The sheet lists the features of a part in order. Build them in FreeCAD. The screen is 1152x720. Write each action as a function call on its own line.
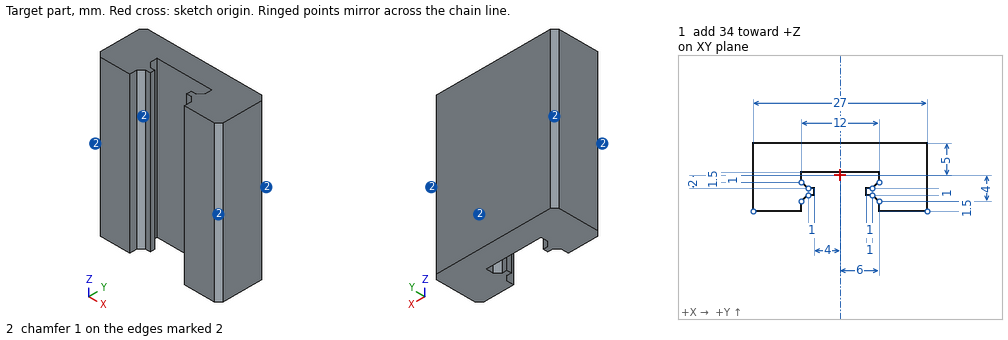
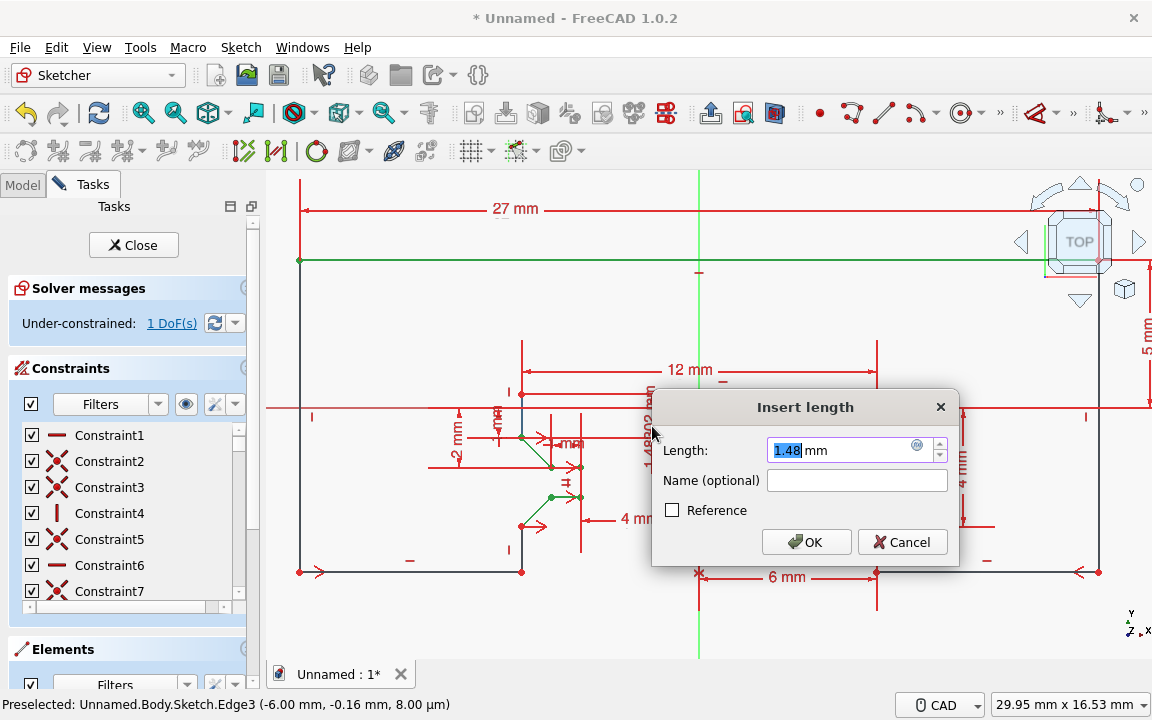
text(1.5)
key(Return)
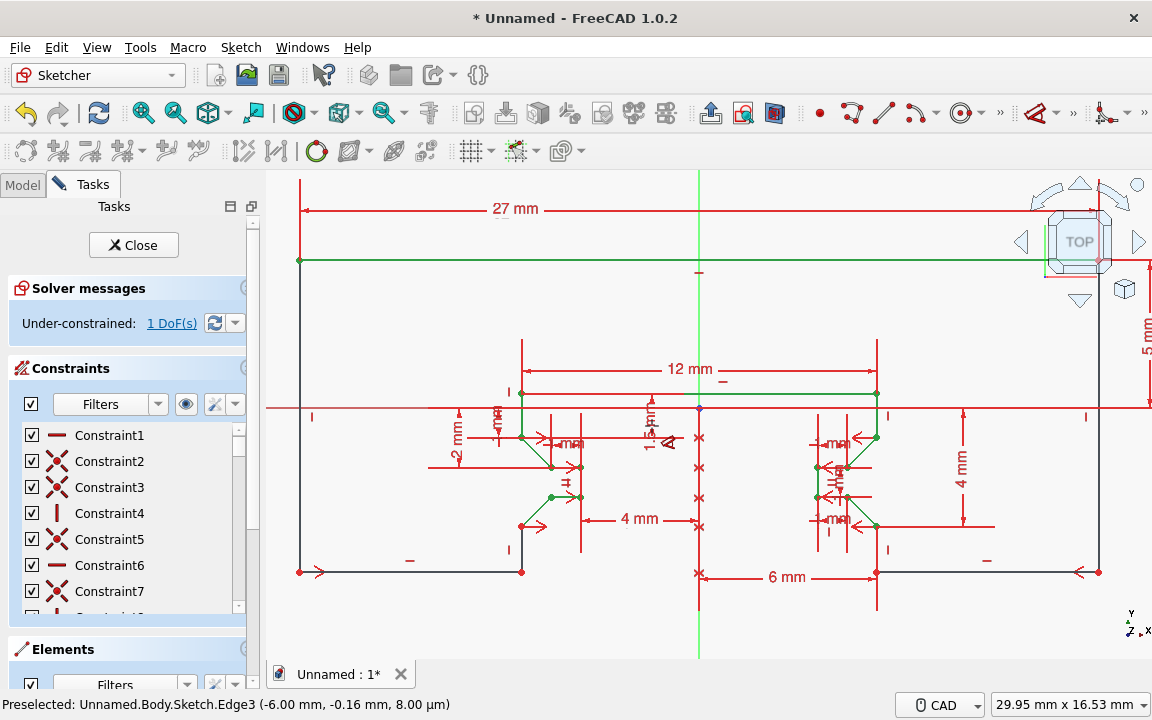
click(877, 540)
click(911, 549)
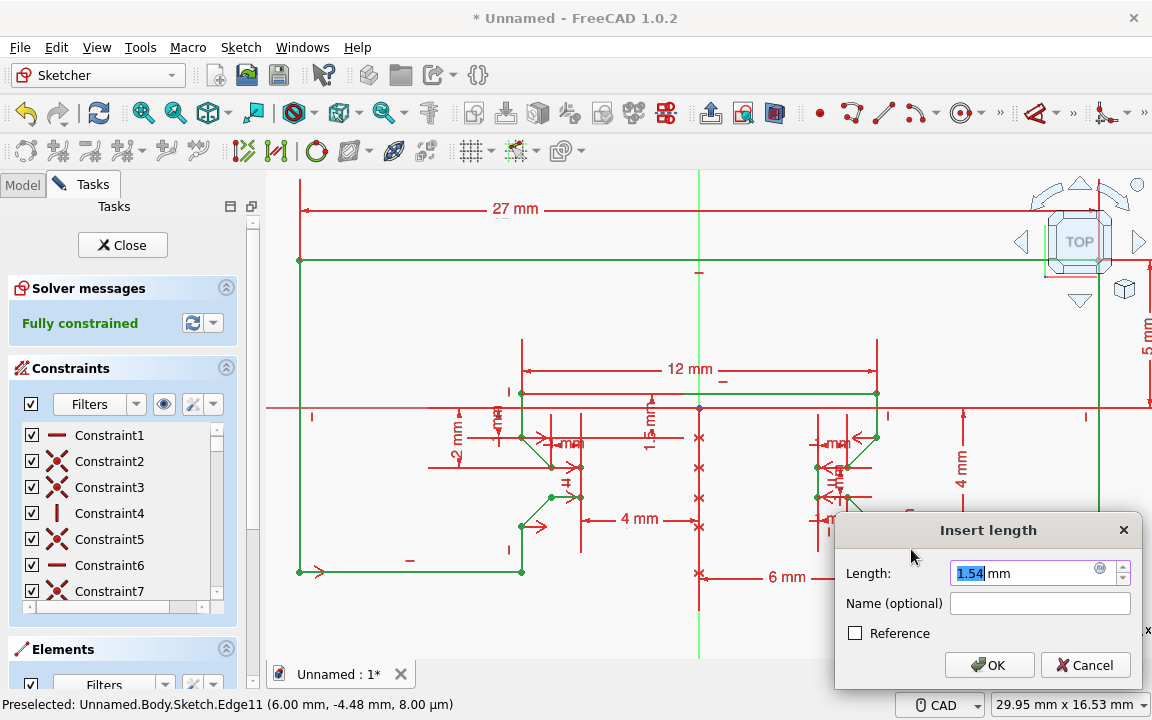
text(1.5)
key(Return)
key(Escape)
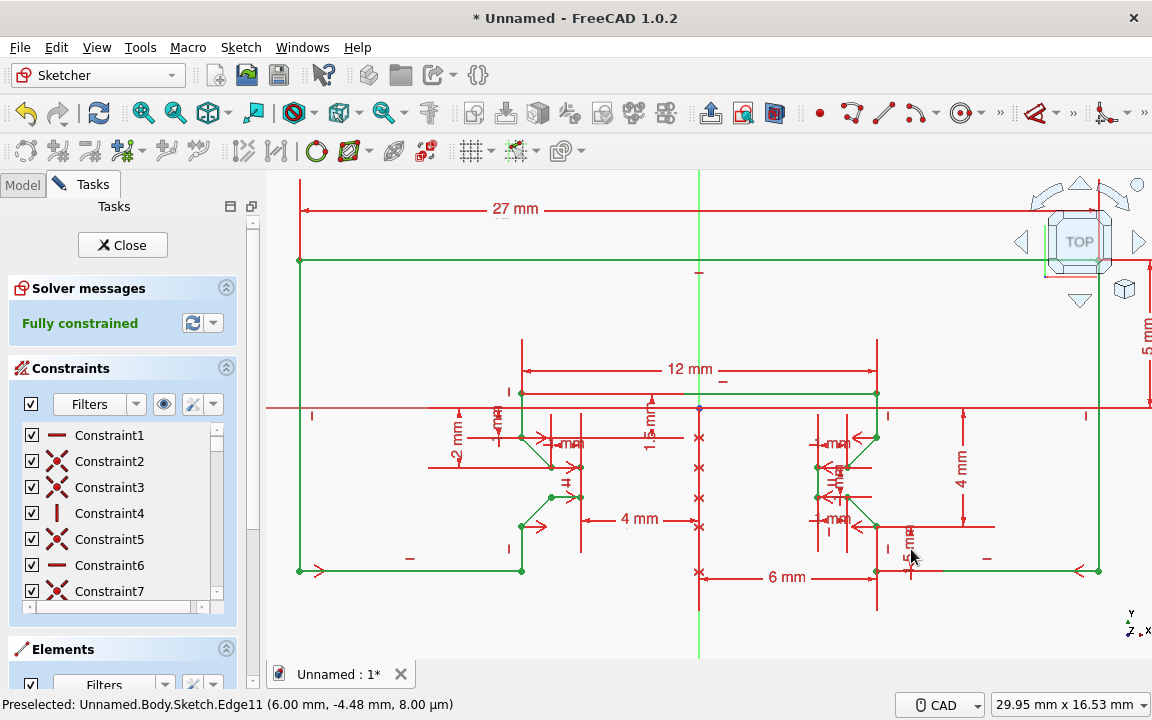
click(123, 245)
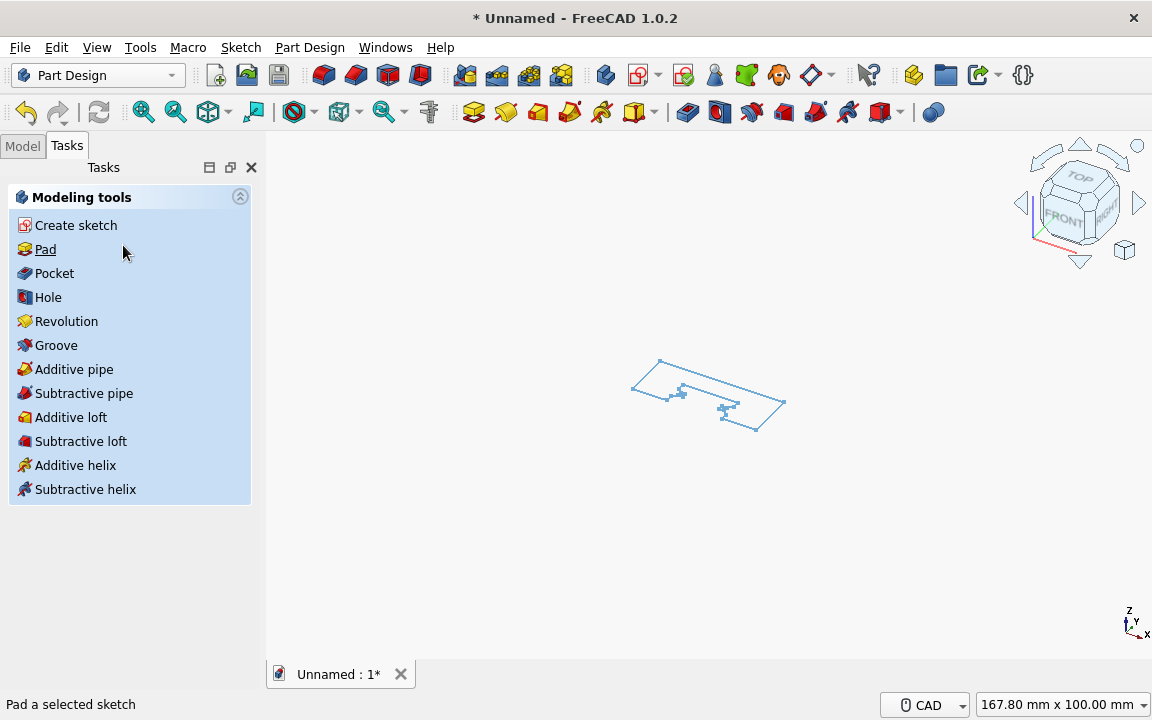
click(474, 112)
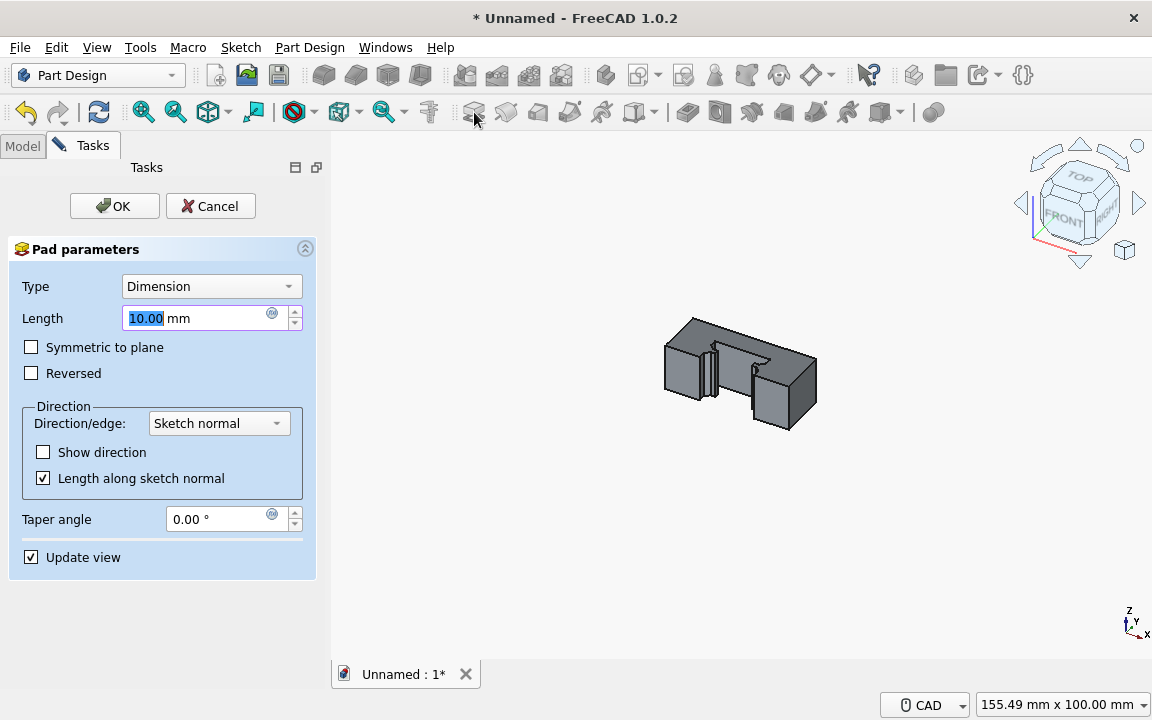
text(34)
key(Tab)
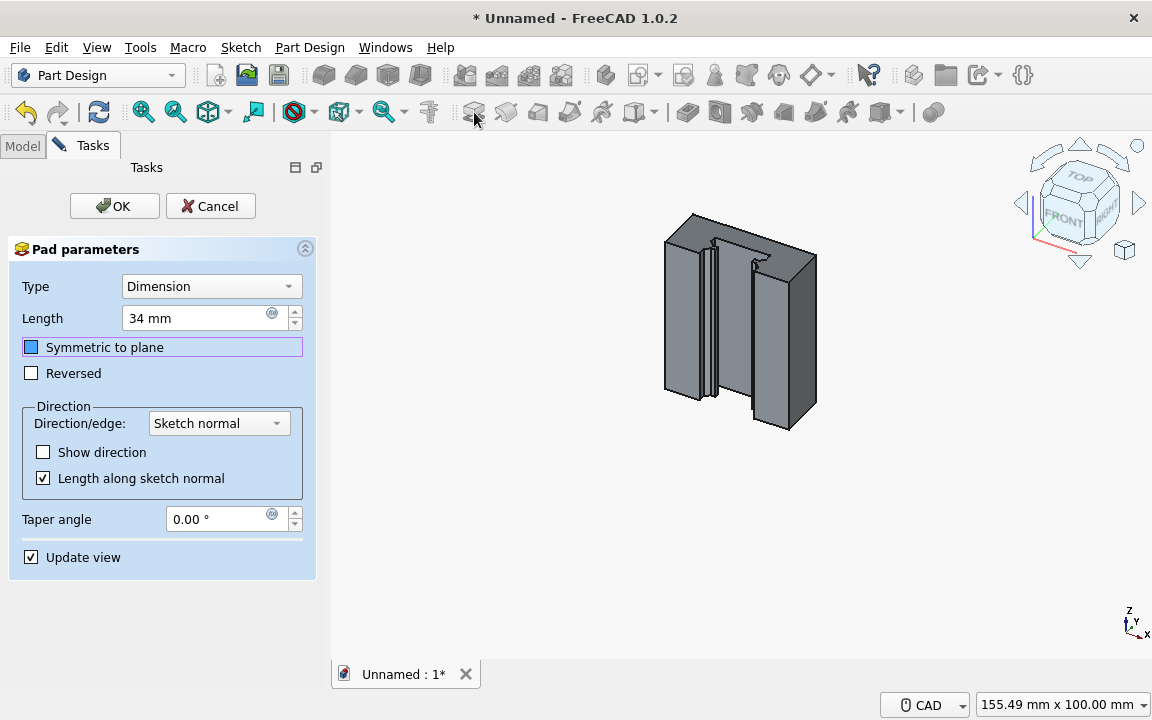
click(115, 206)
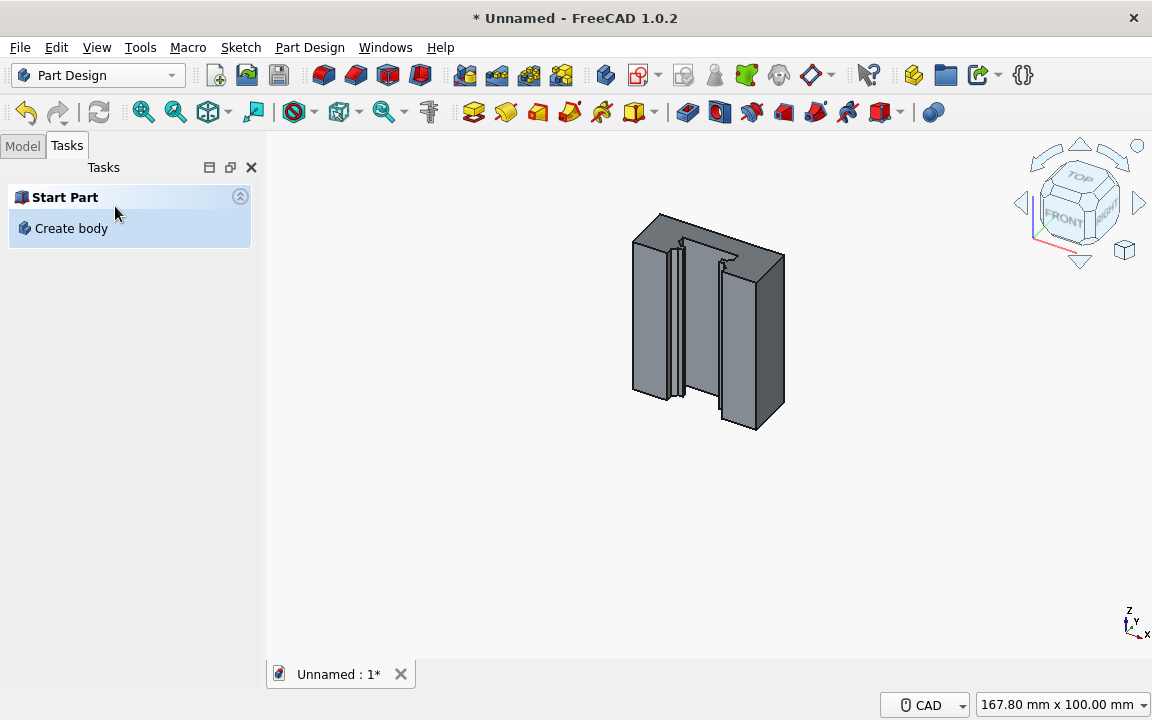
click(144, 112)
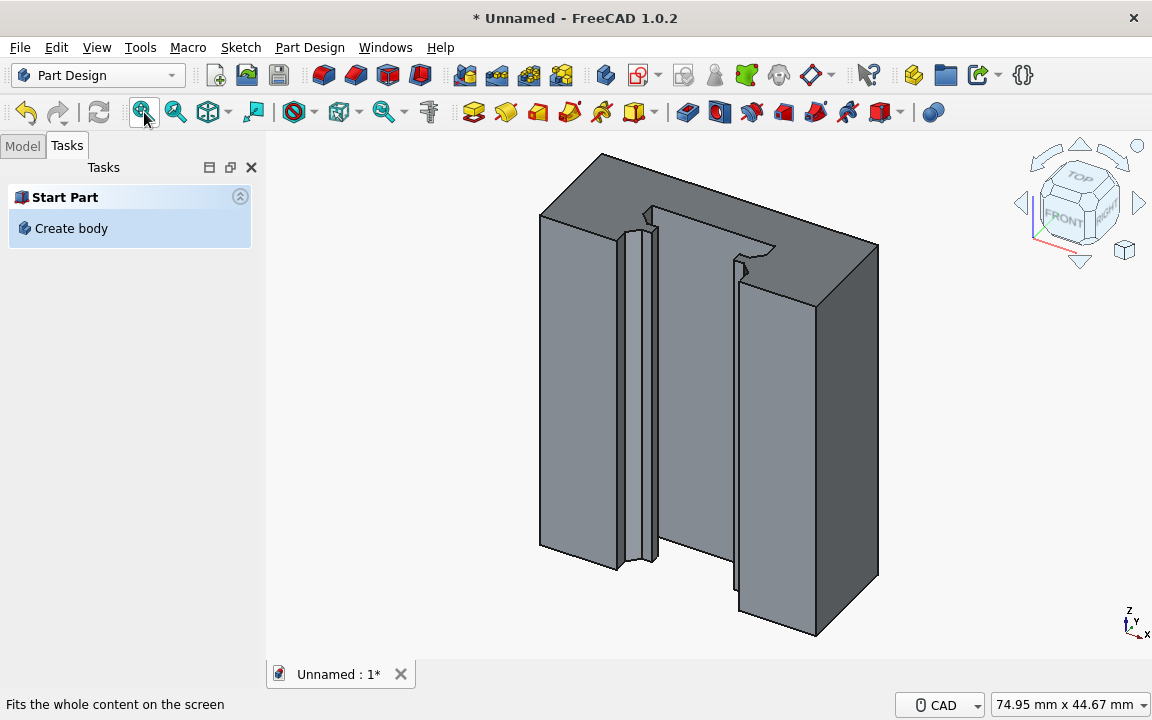
click(816, 471)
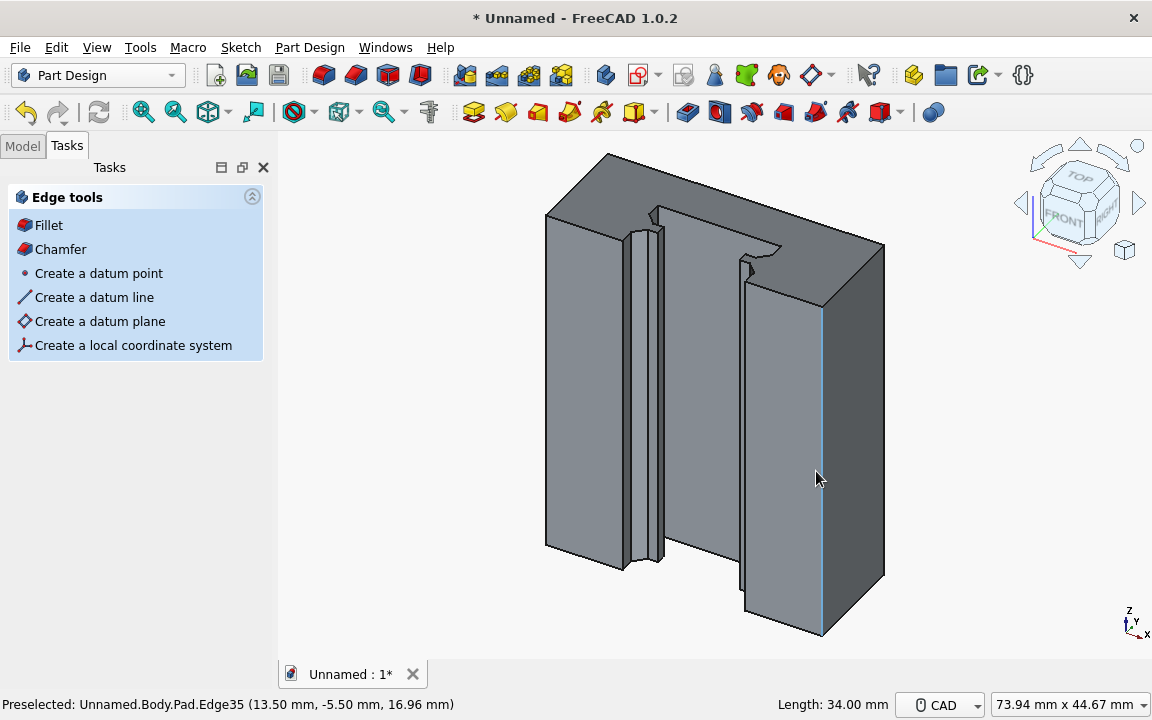
key(0)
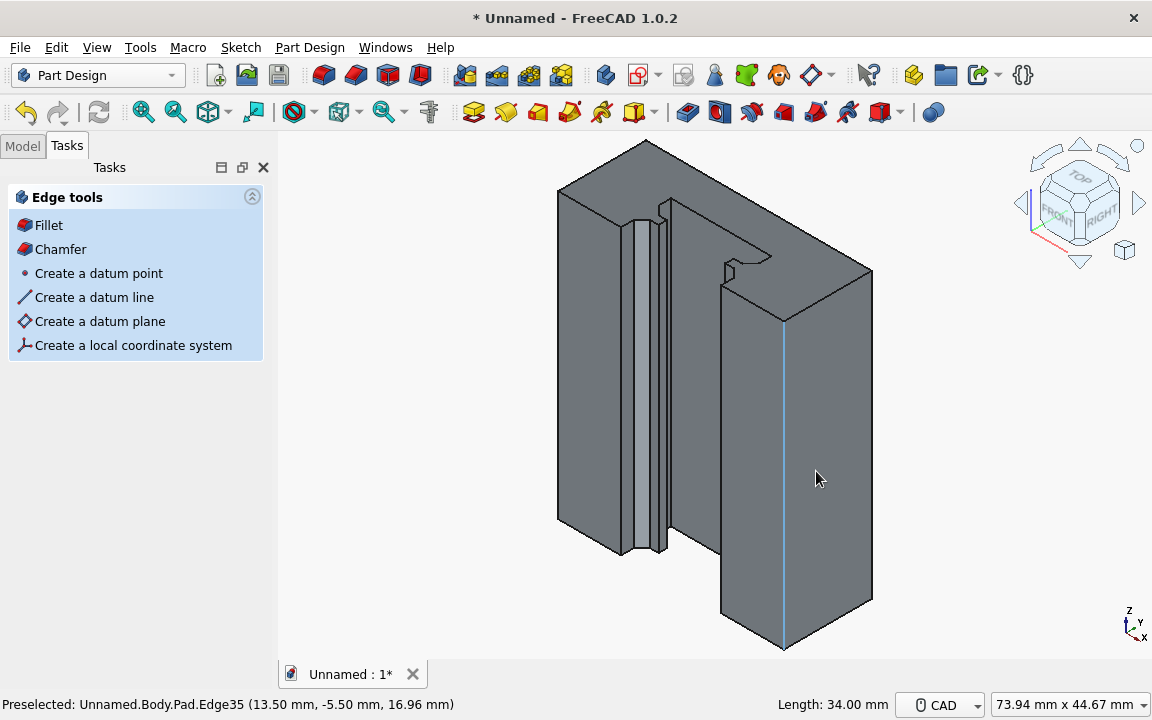
key(2)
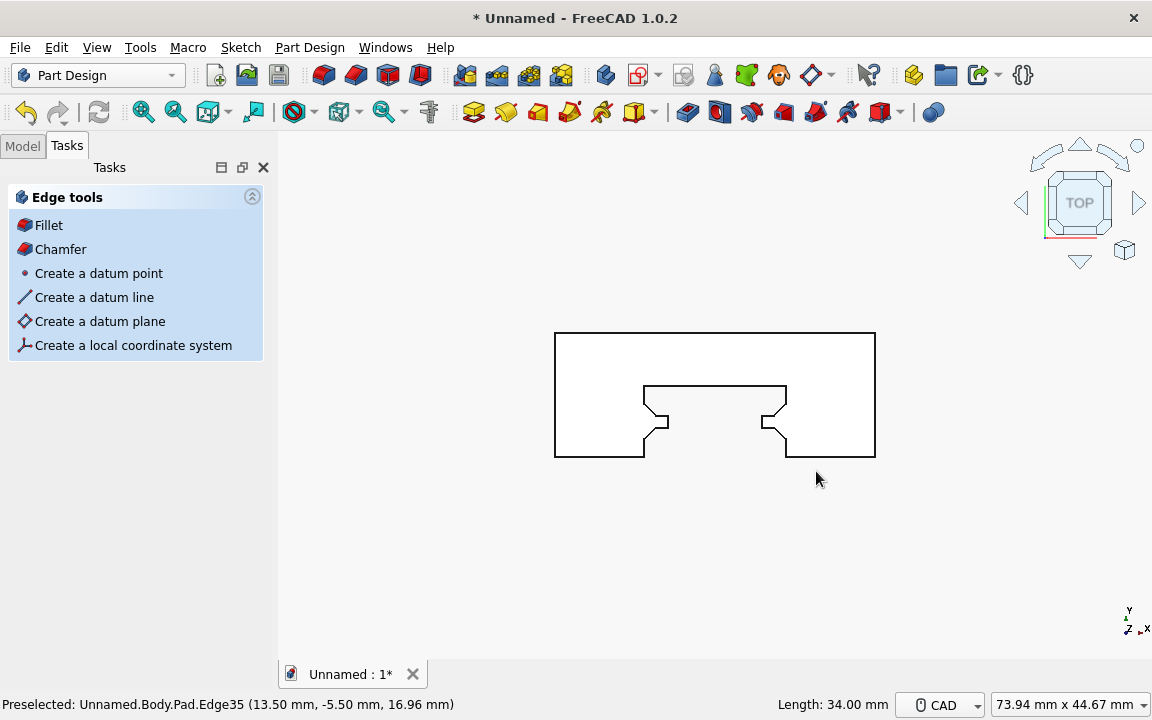
click(144, 112)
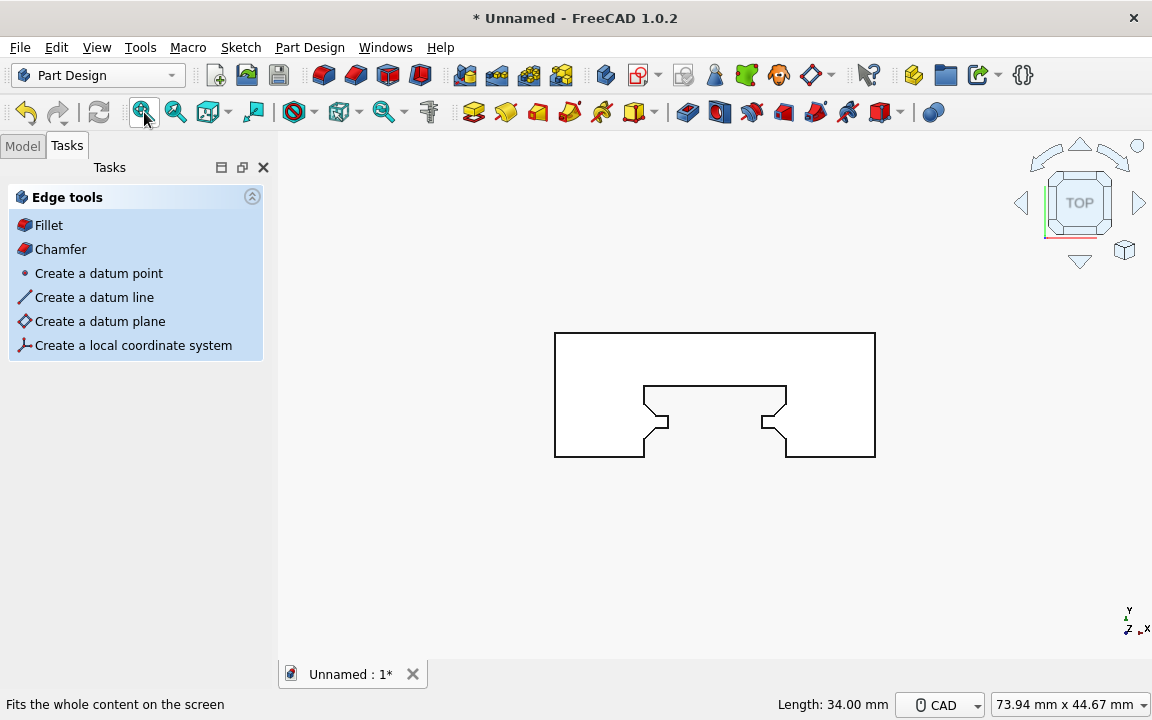
key(1)